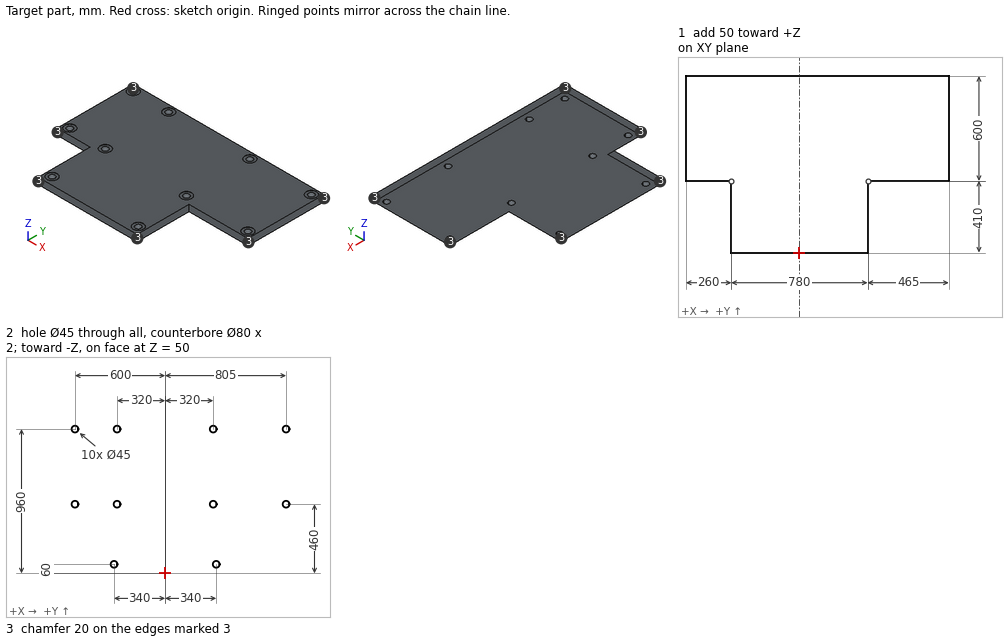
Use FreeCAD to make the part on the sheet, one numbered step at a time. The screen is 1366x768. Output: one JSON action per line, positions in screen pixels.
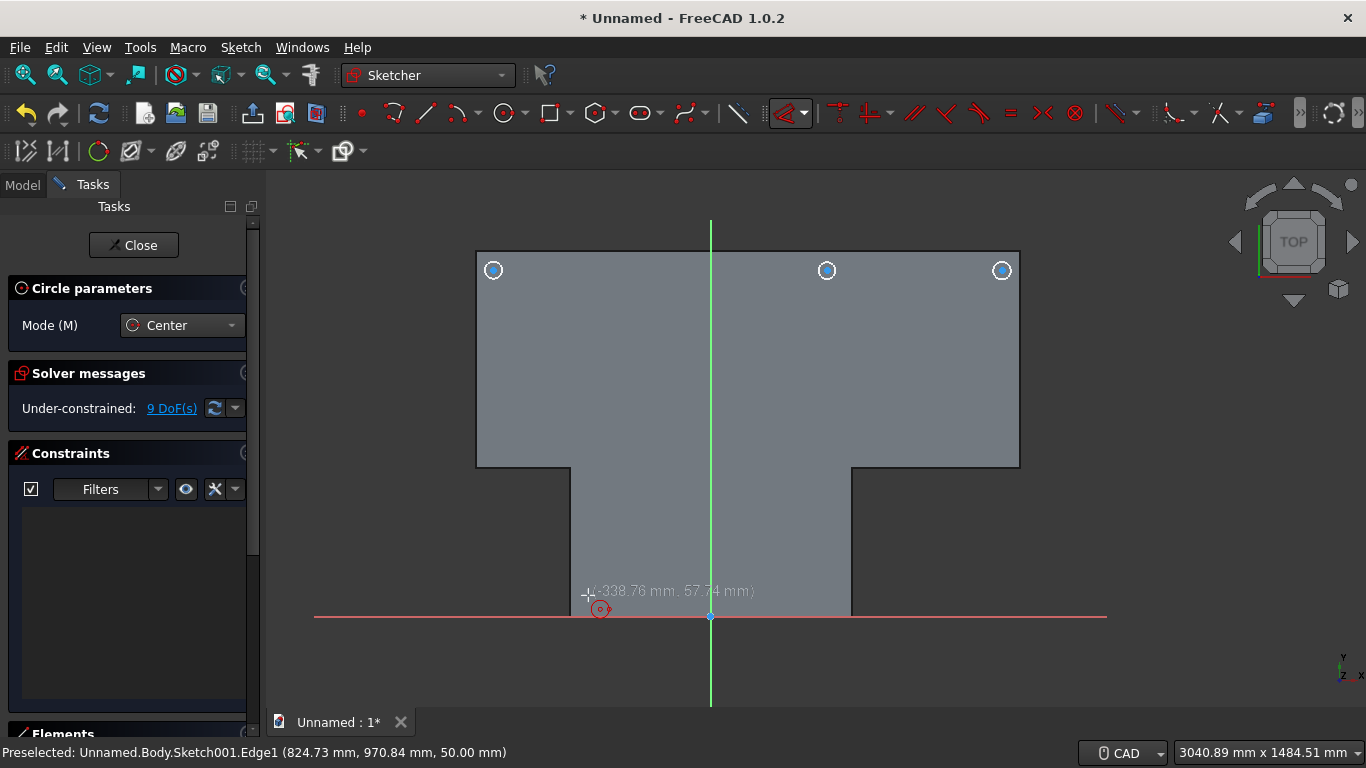
{"action": "left_click", "coordinate": [588, 595]}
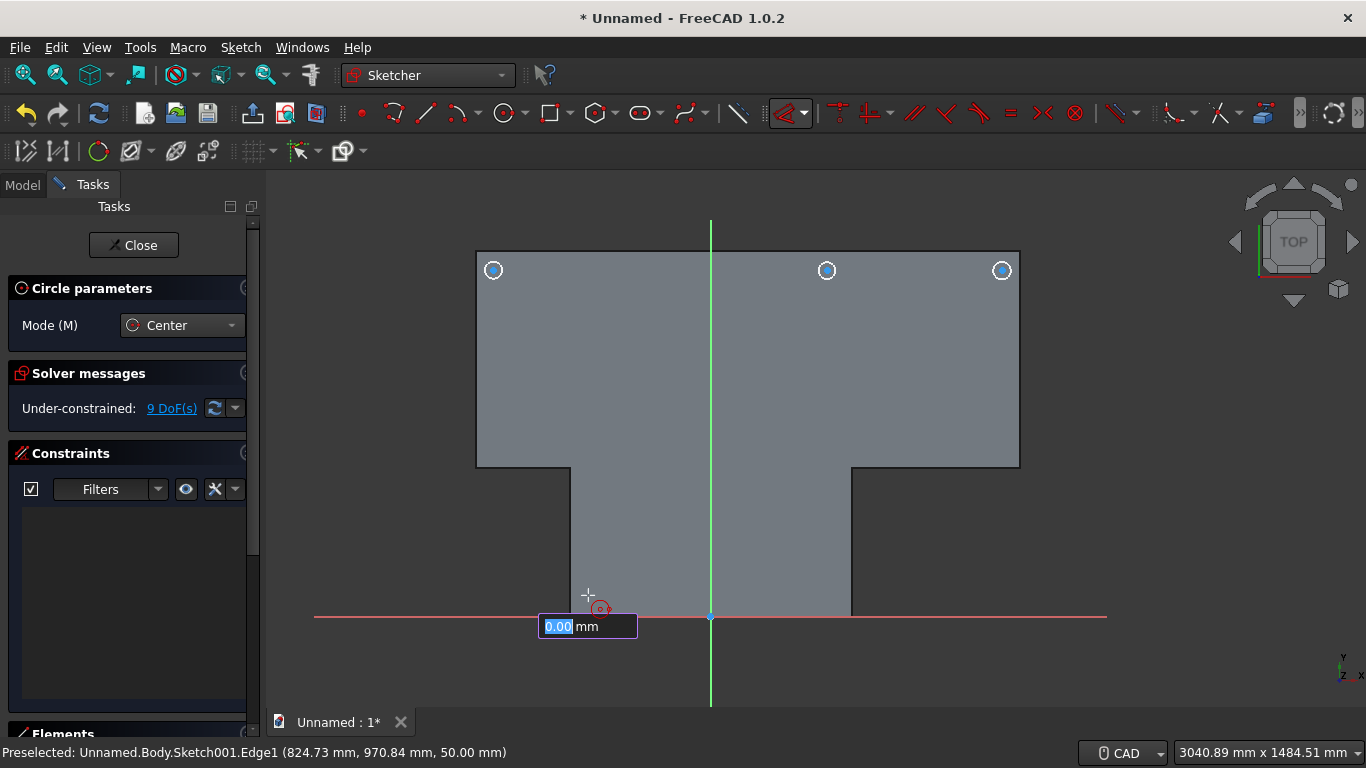
{"action": "scroll", "coordinate": [594, 589], "scroll_direction": "up", "scroll_amount": 4}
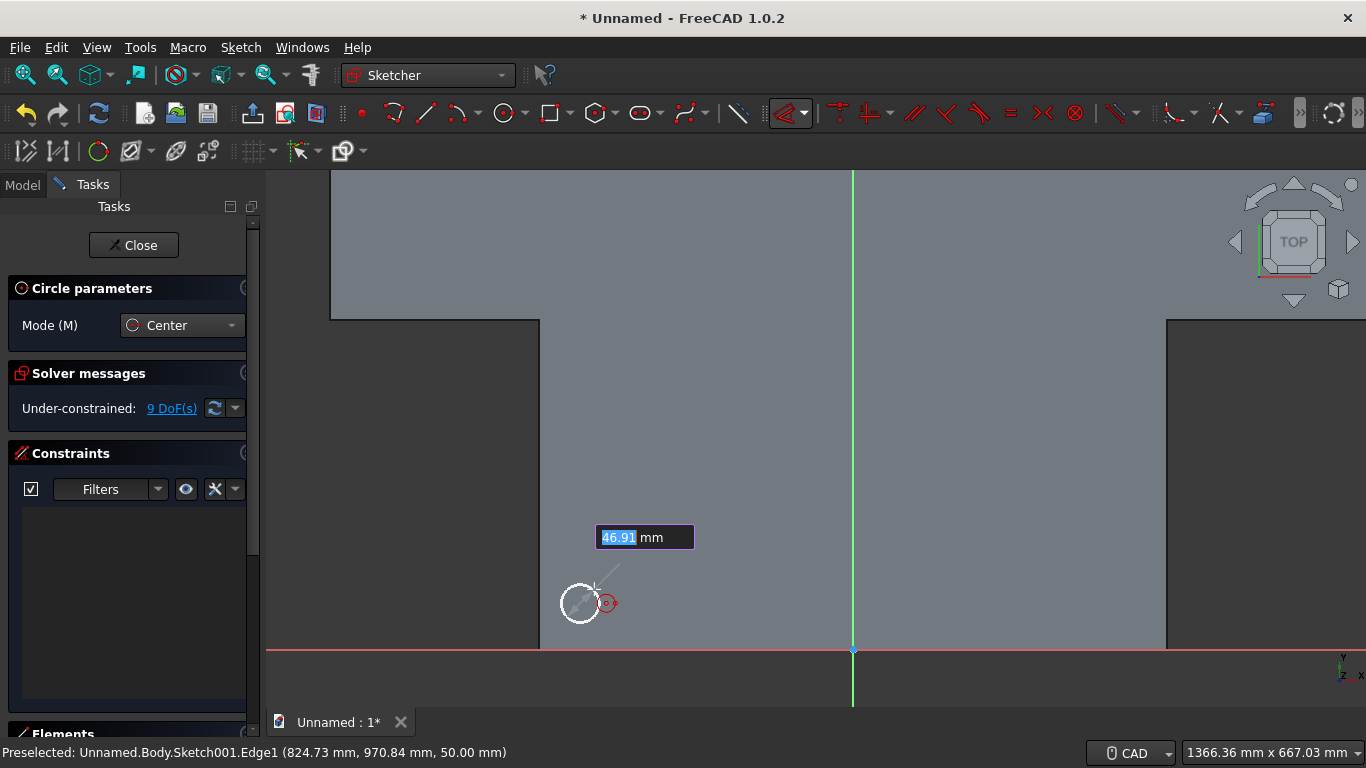
{"action": "left_click", "coordinate": [593, 589]}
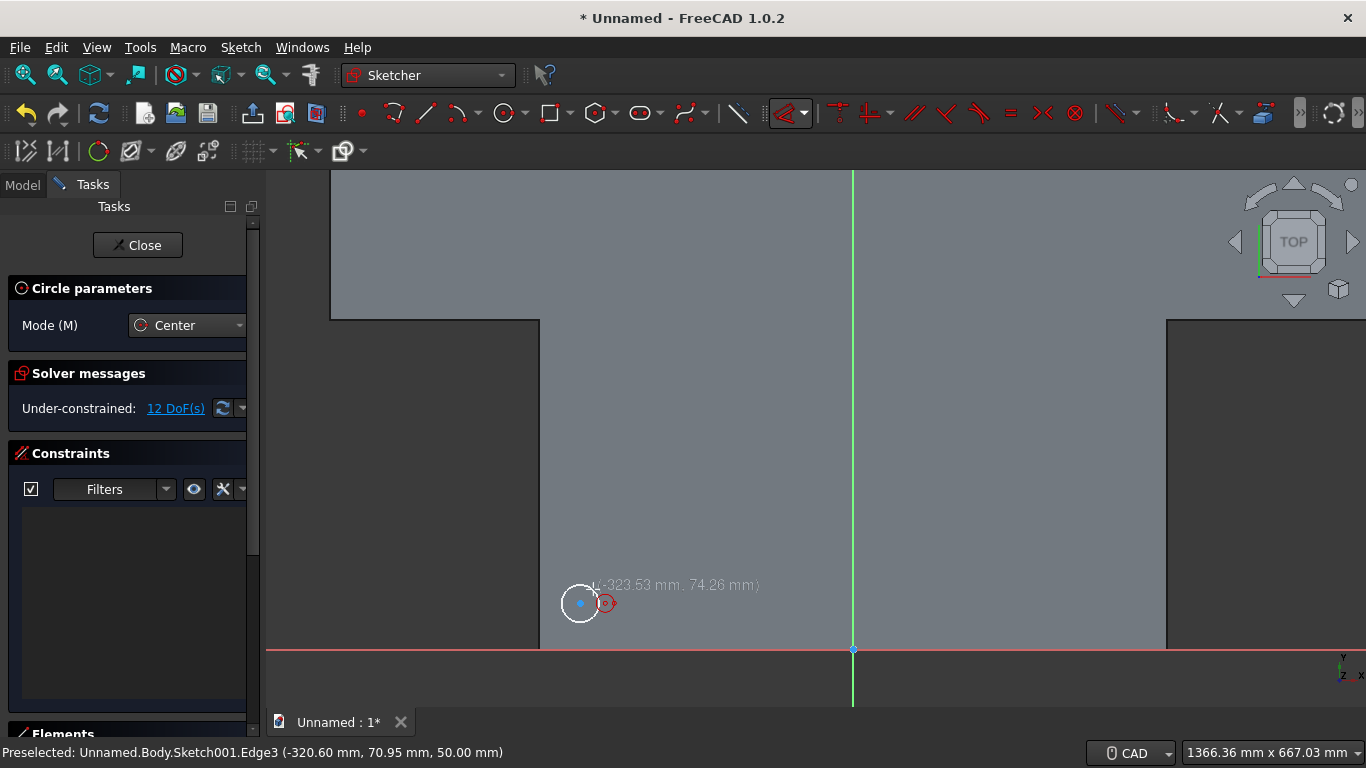
{"action": "scroll", "coordinate": [1127, 601], "scroll_direction": "up", "scroll_amount": 2}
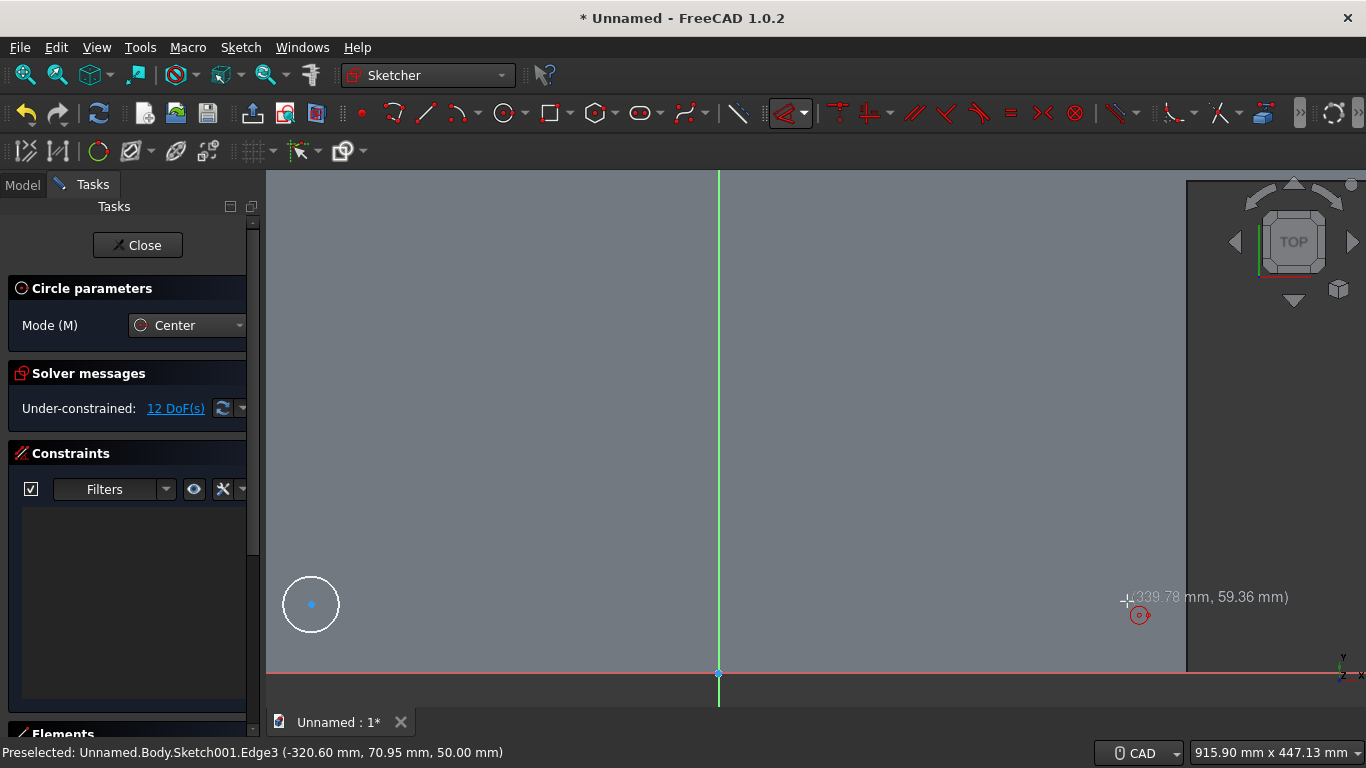
{"action": "scroll", "coordinate": [707, 592], "scroll_direction": "down", "scroll_amount": 6}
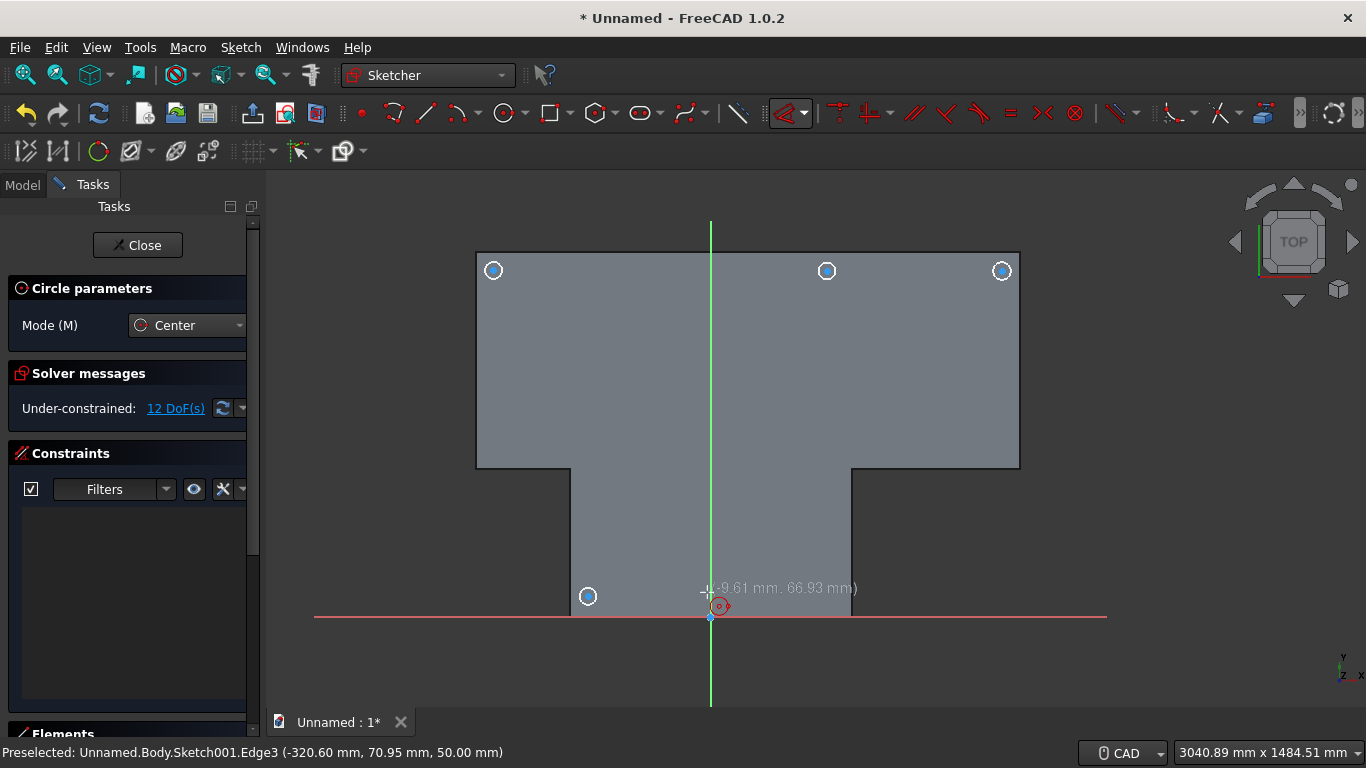
{"action": "left_click", "coordinate": [834, 595]}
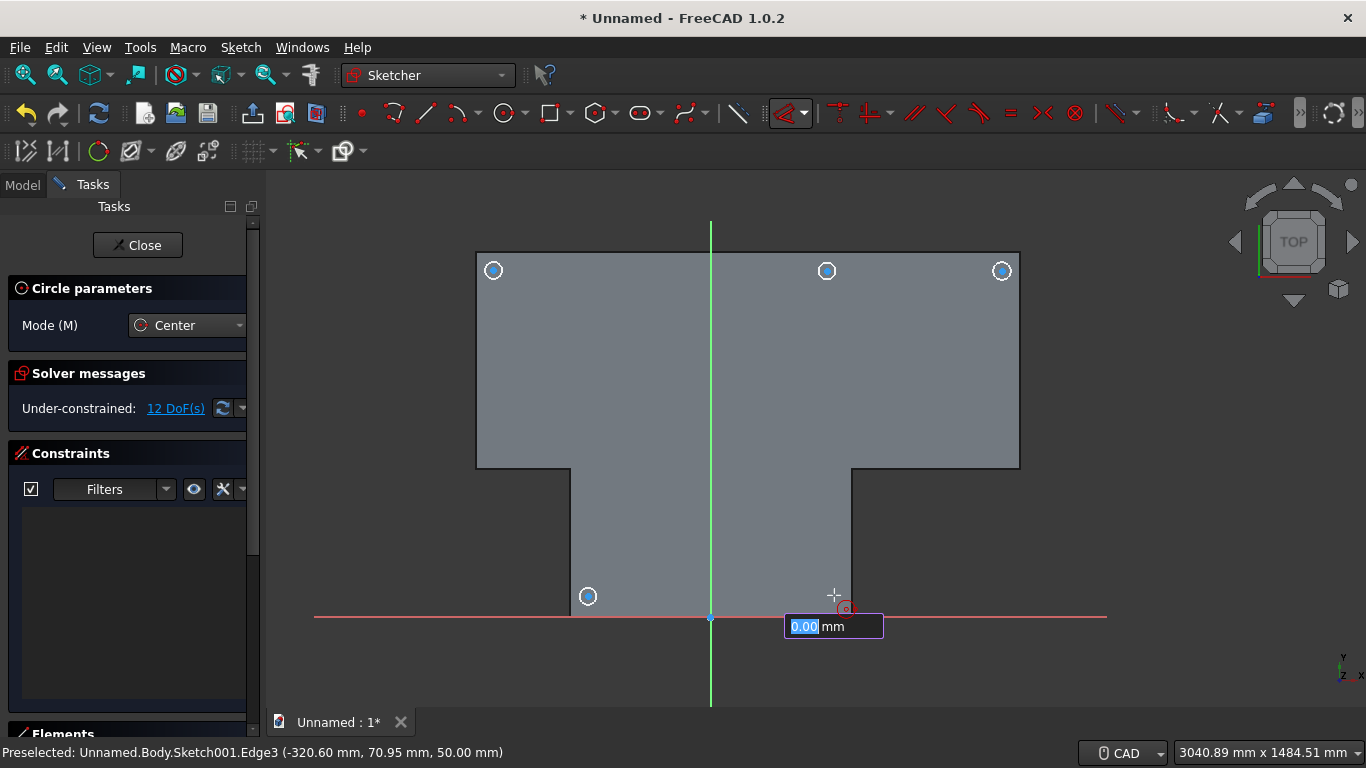
{"action": "scroll", "coordinate": [840, 590], "scroll_direction": "up", "scroll_amount": 4}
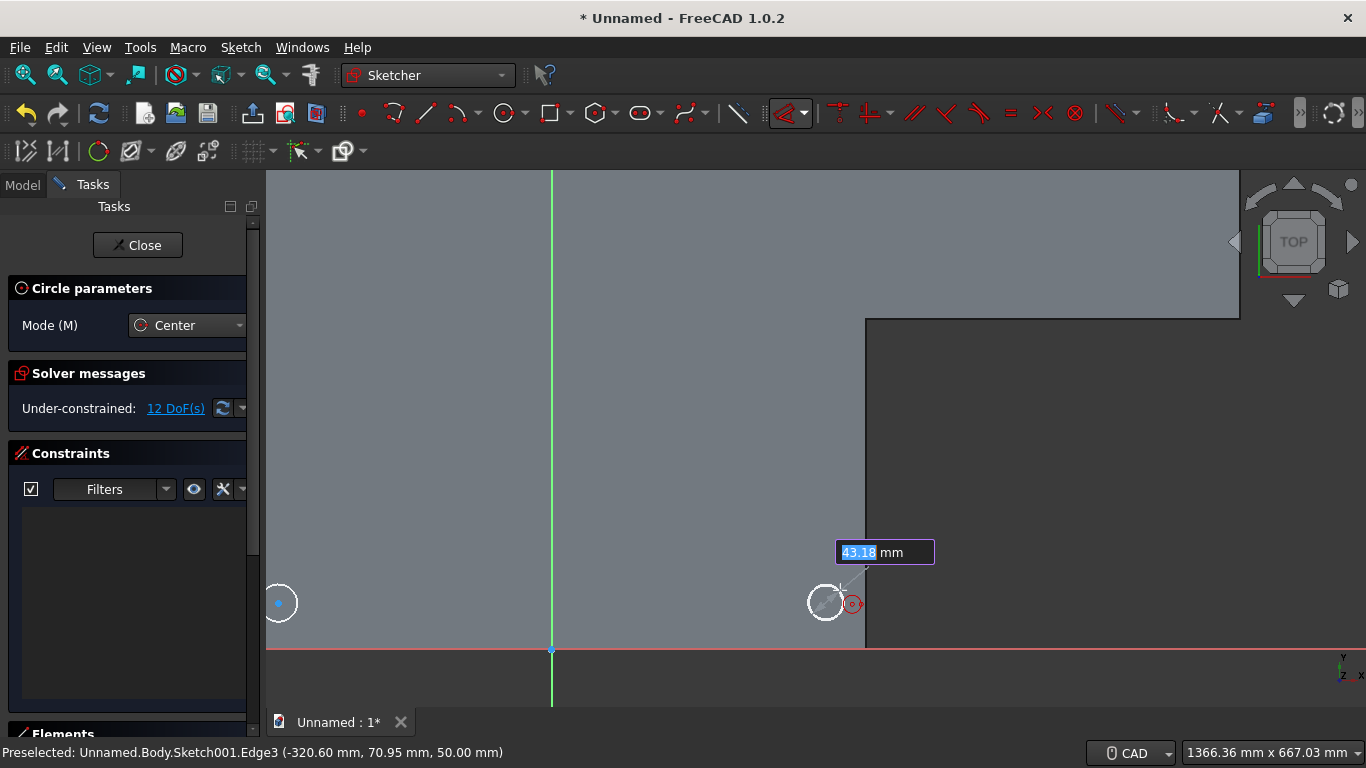
{"action": "left_click", "coordinate": [838, 588]}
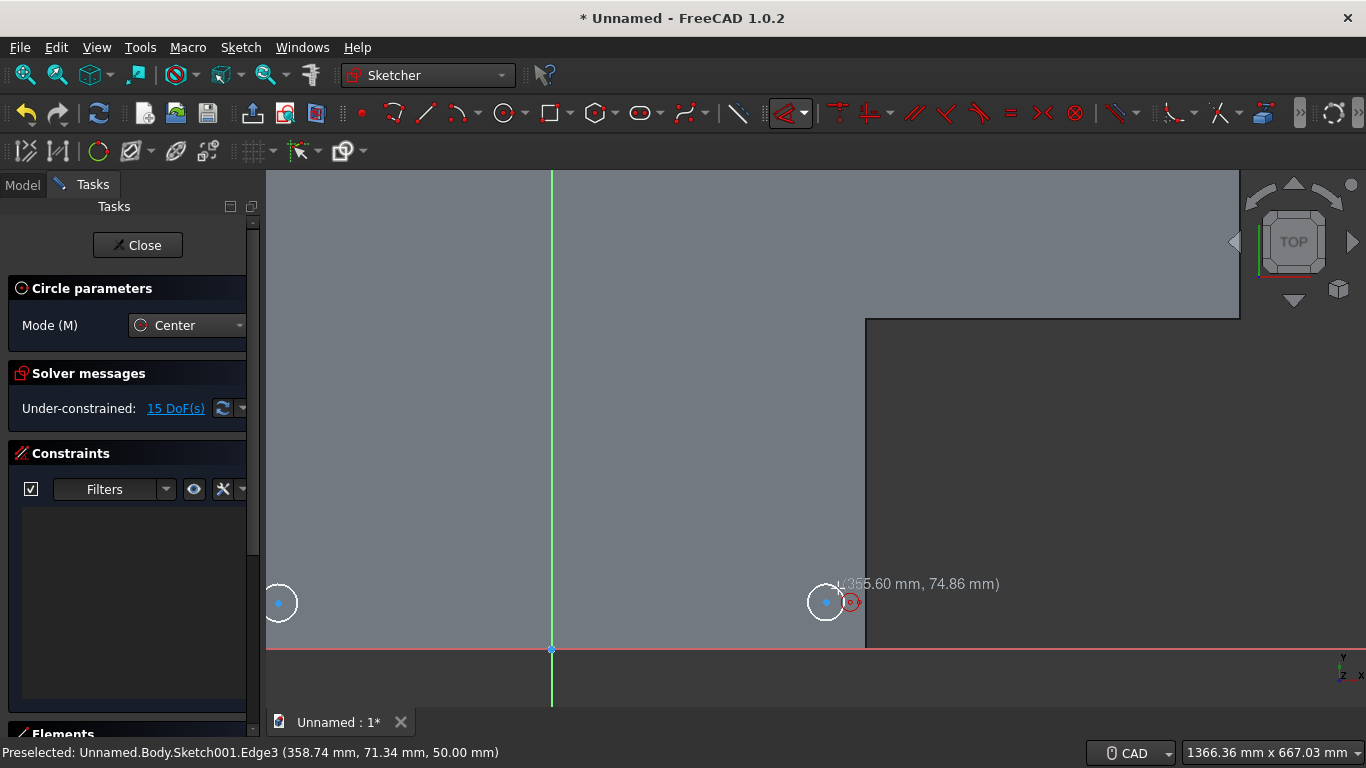
{"action": "scroll", "coordinate": [840, 589], "scroll_direction": "down", "scroll_amount": 4}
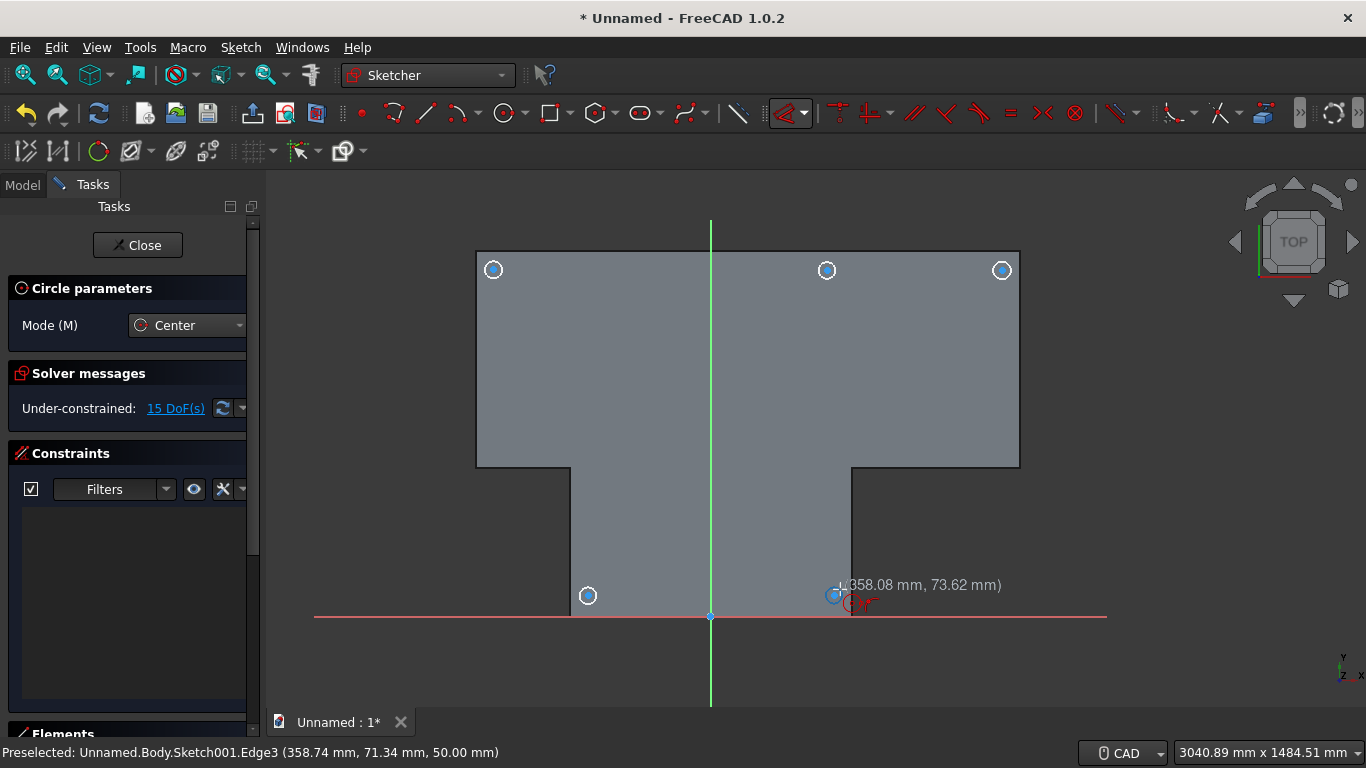
{"action": "scroll", "coordinate": [595, 269], "scroll_direction": "up", "scroll_amount": 6}